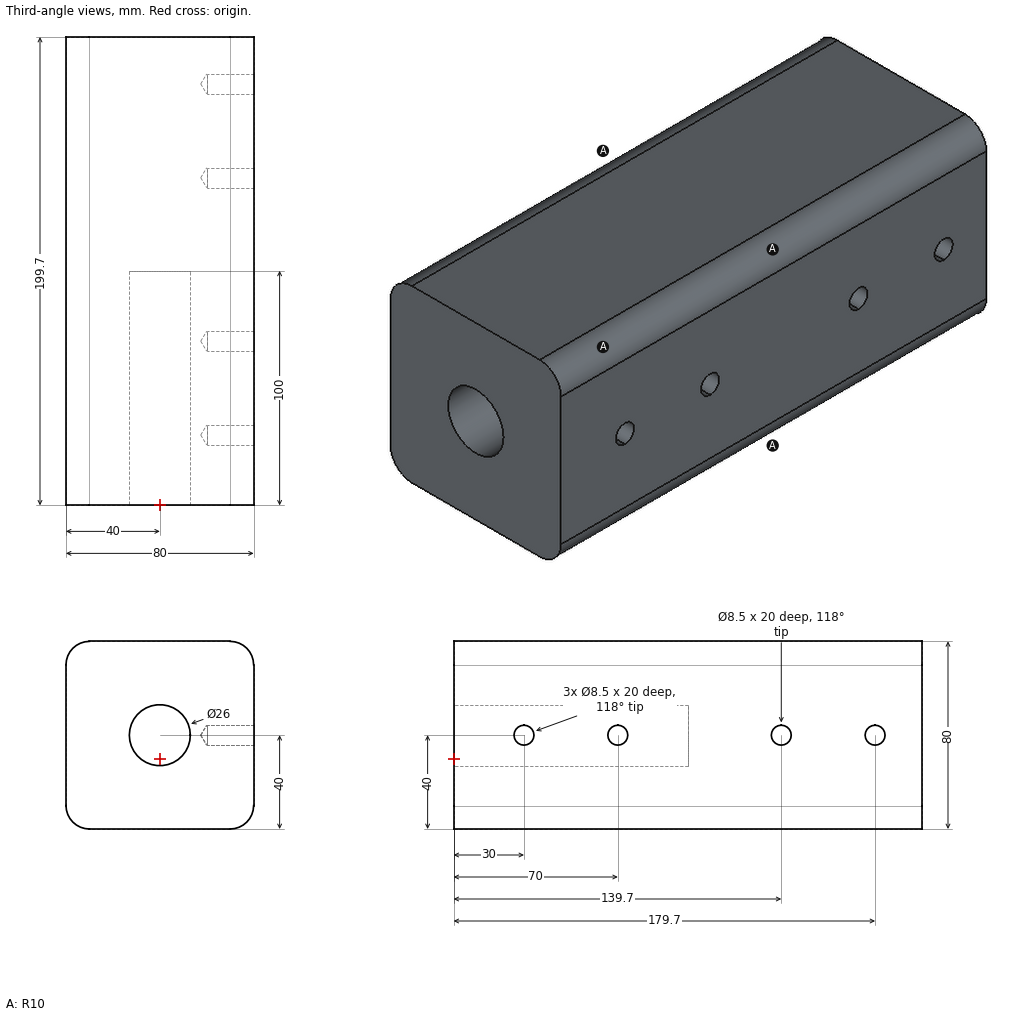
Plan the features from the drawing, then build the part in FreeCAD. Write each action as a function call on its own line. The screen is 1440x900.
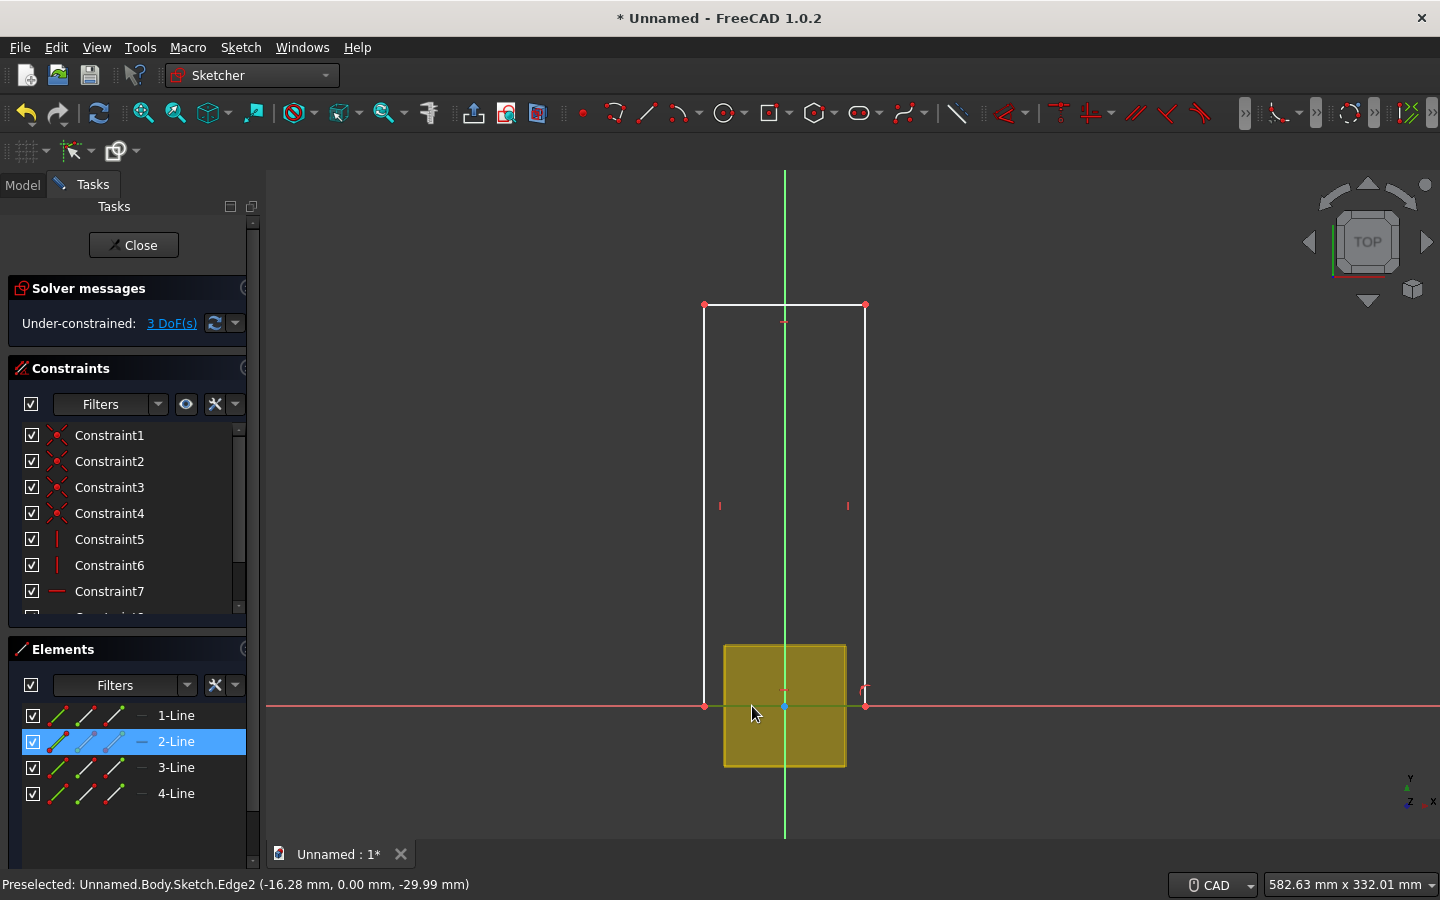
key(l)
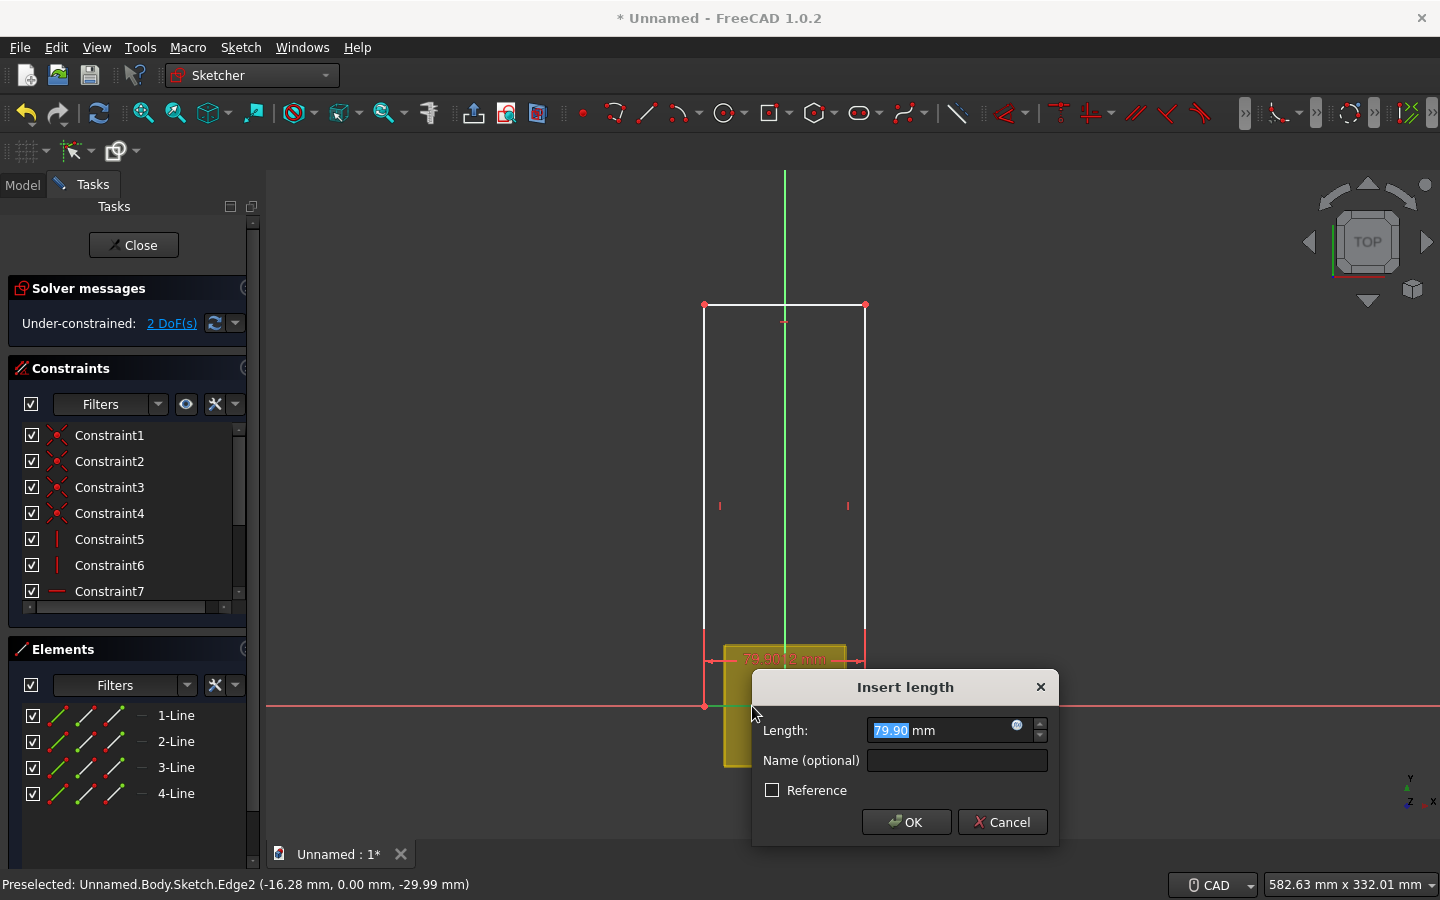
text(80)
key(Return)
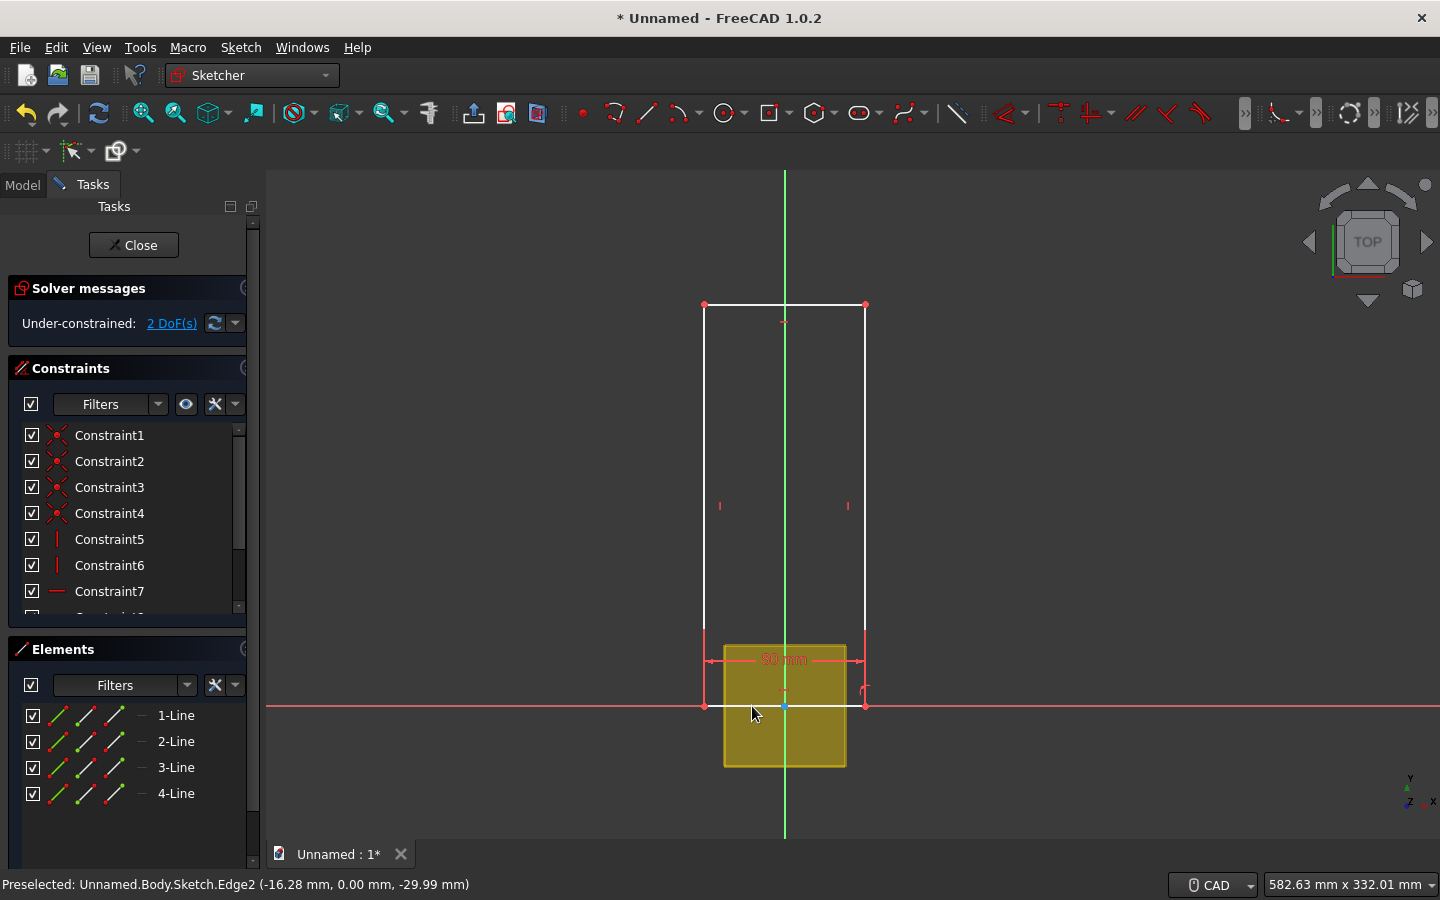
click(704, 305)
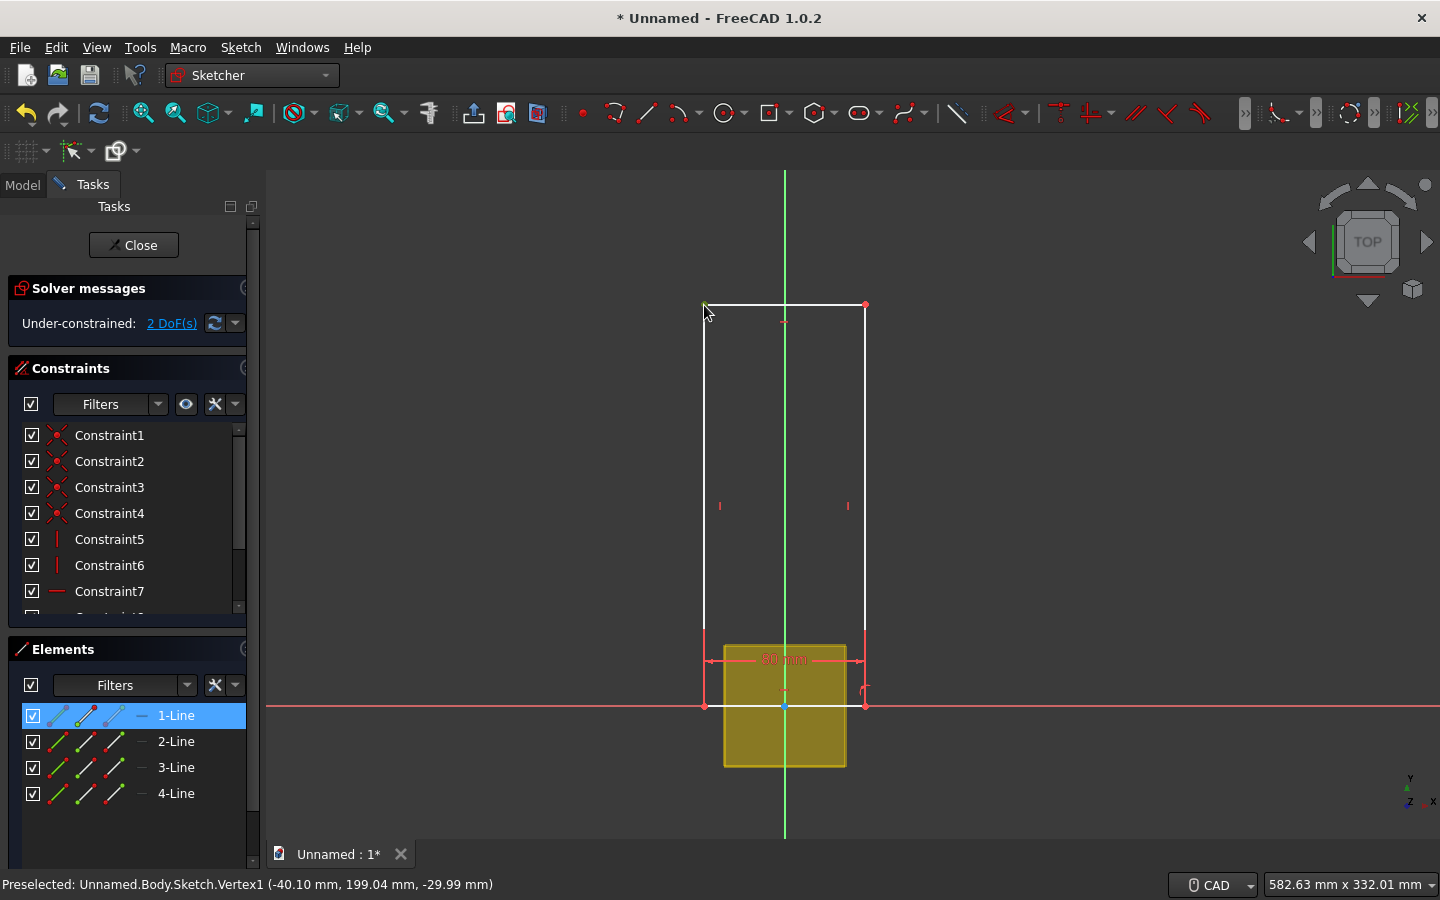
click(1028, 114)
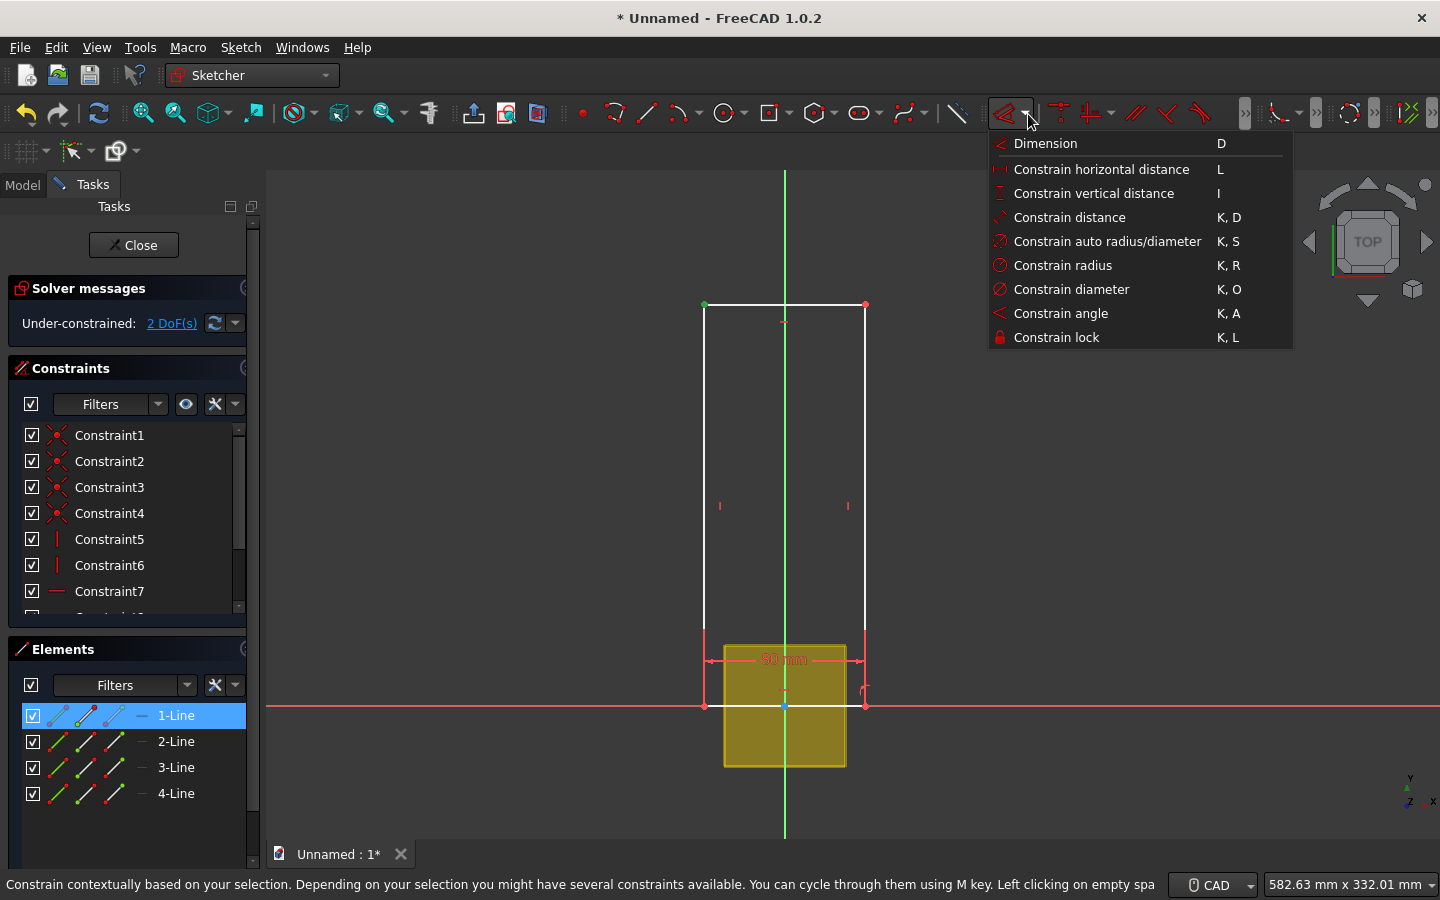
click(1141, 169)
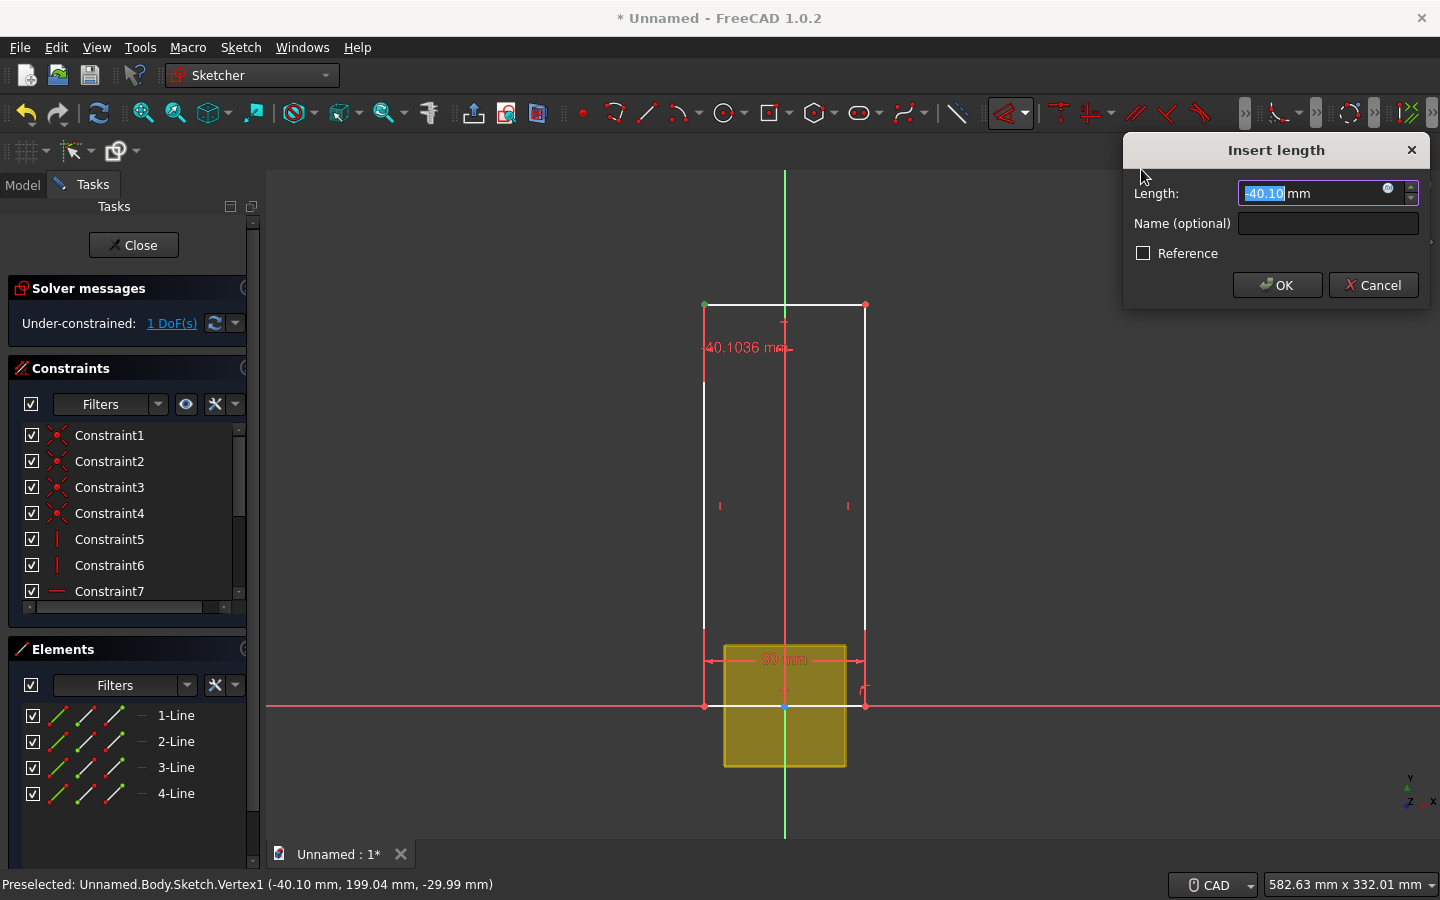
text(-40)
key(Return)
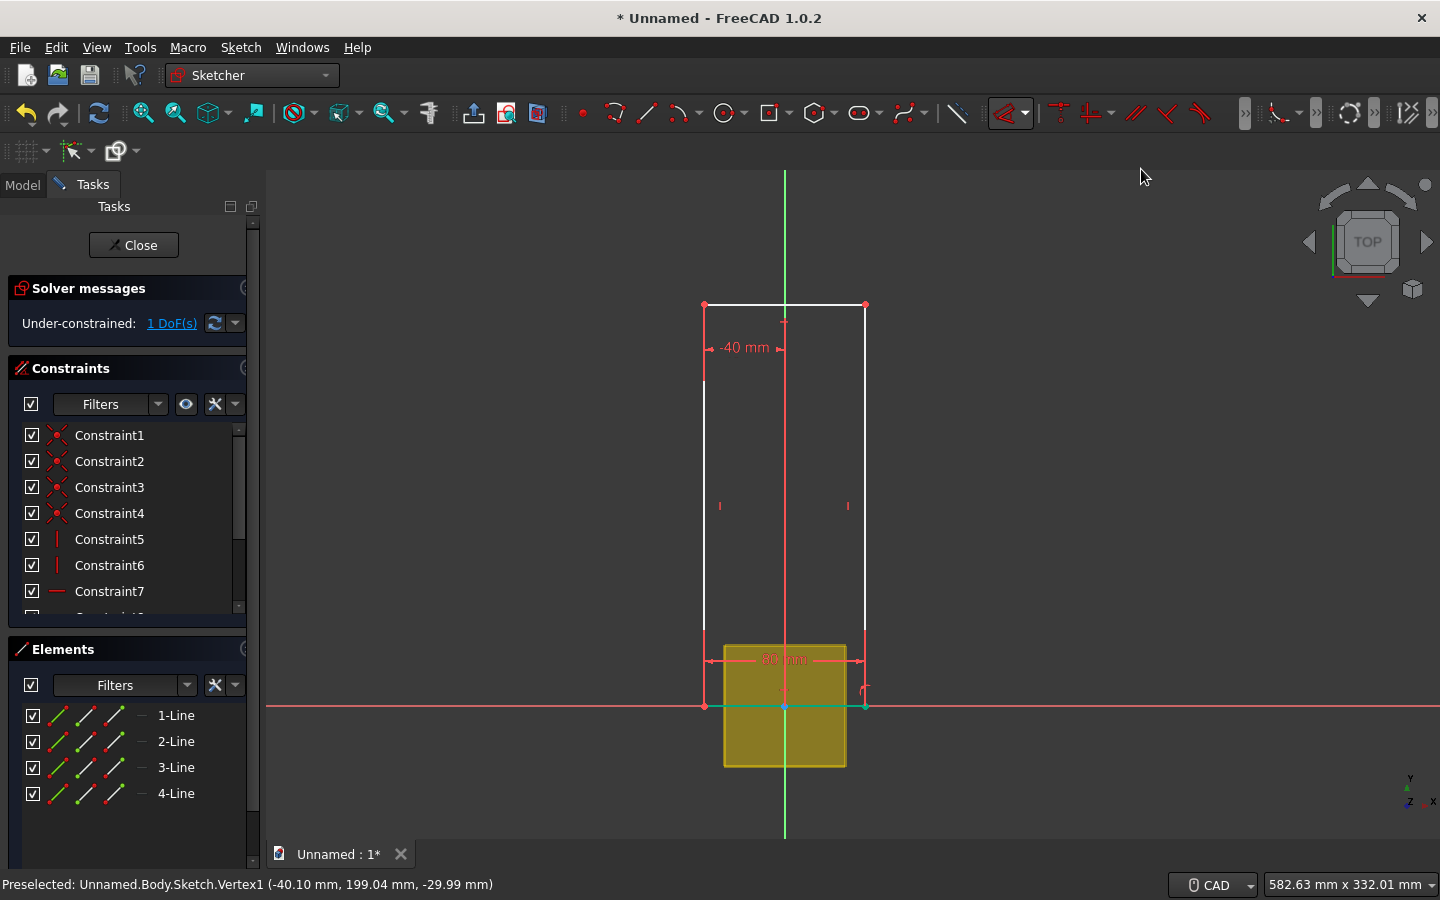
click(704, 425)